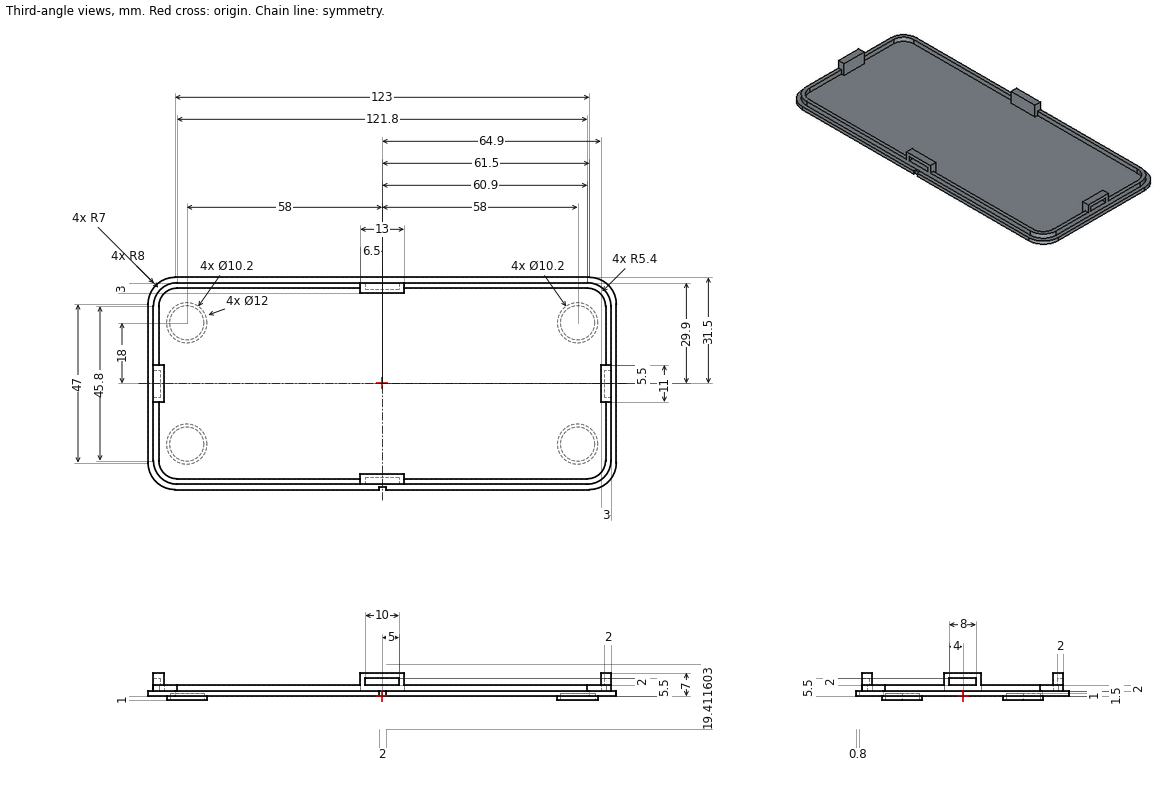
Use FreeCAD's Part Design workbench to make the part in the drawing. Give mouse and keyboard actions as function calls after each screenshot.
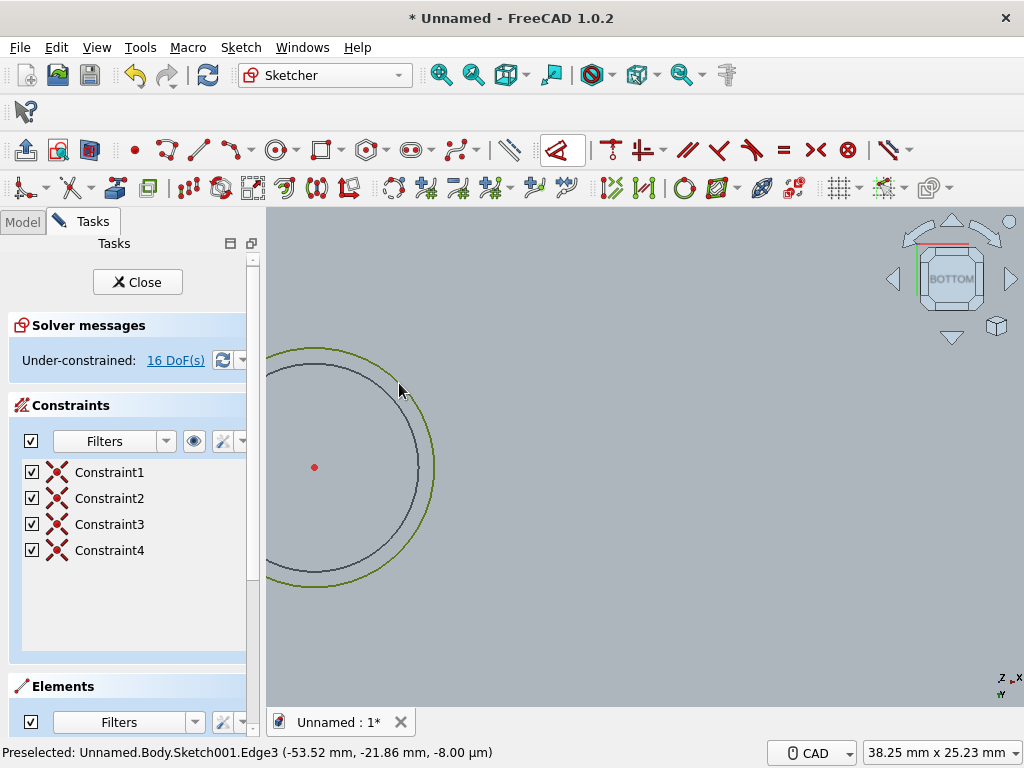
scroll(401, 385, down, 9)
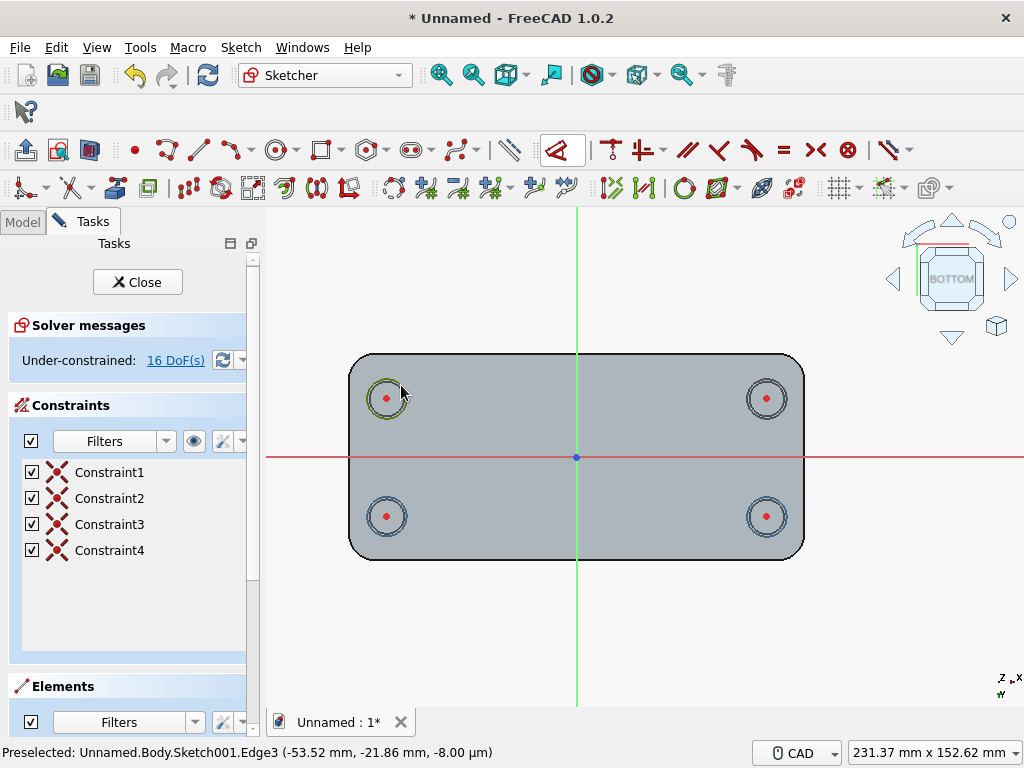
scroll(781, 385, up, 9)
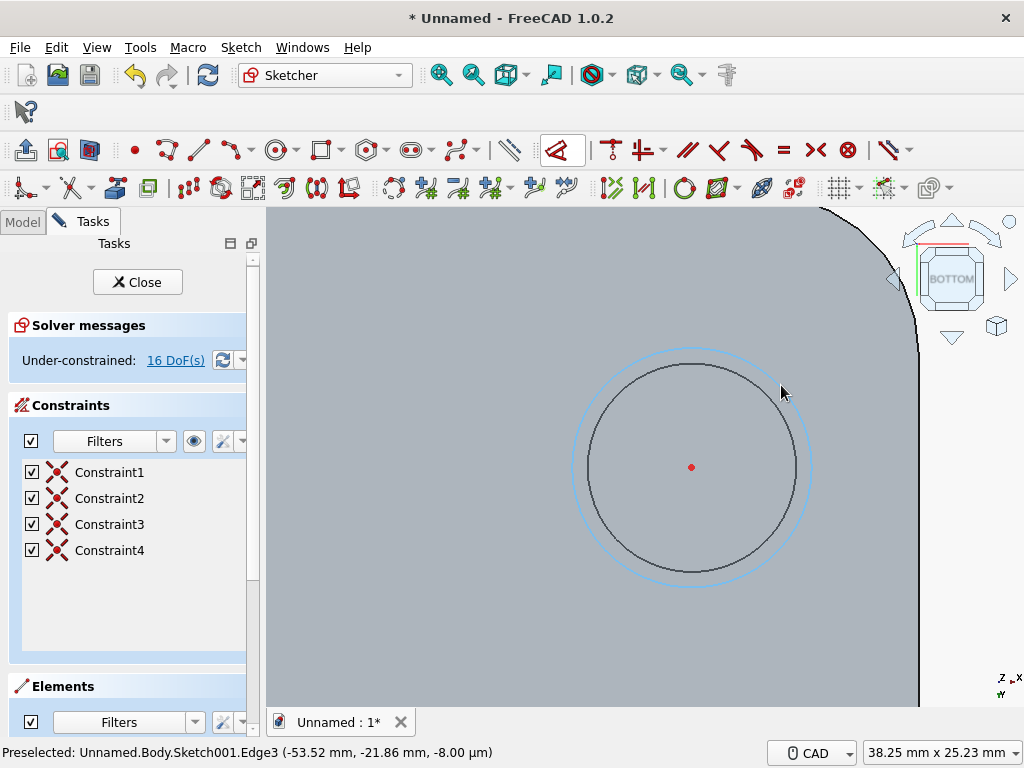
click(776, 383)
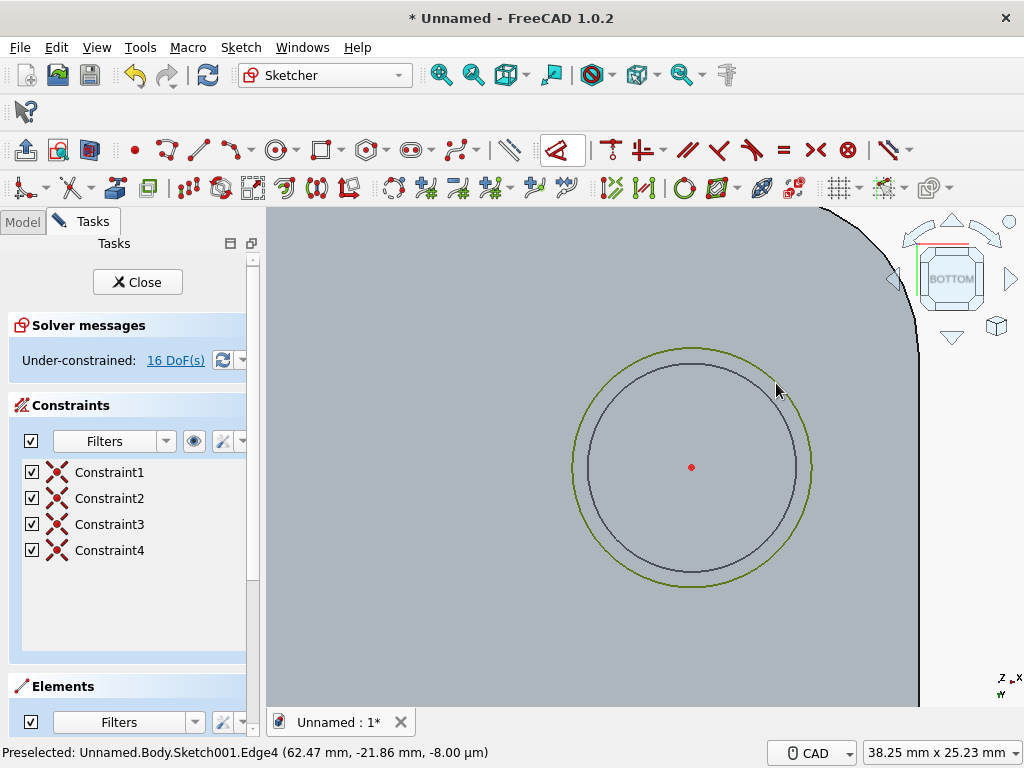
key(e)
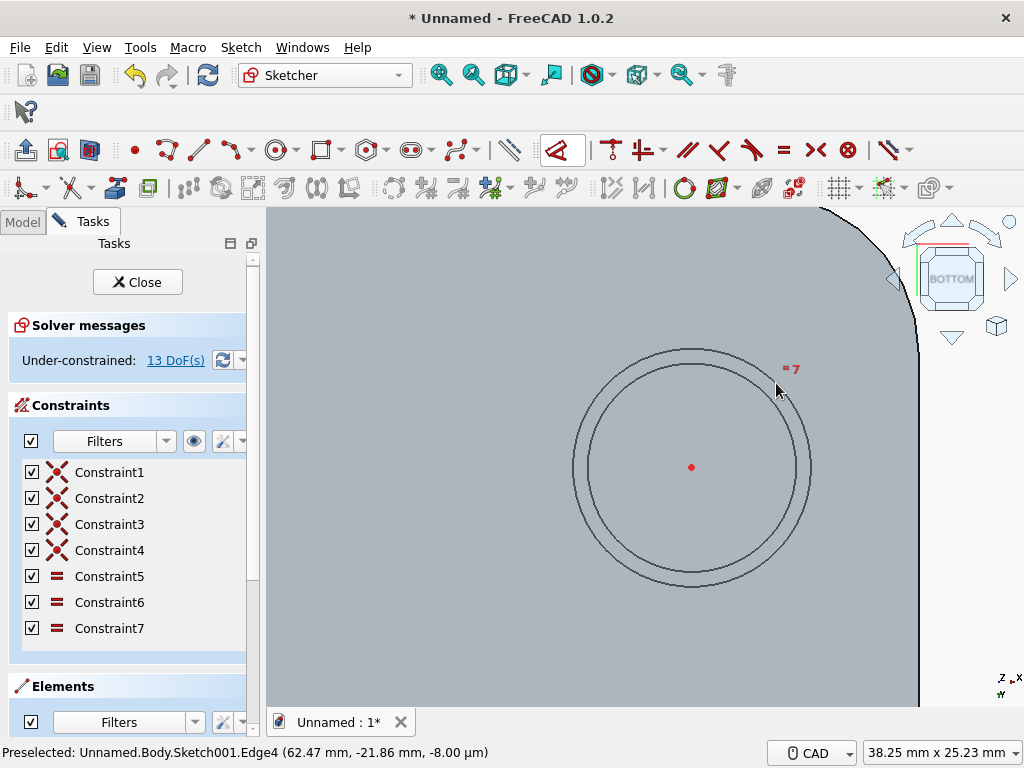
scroll(782, 385, down, 9)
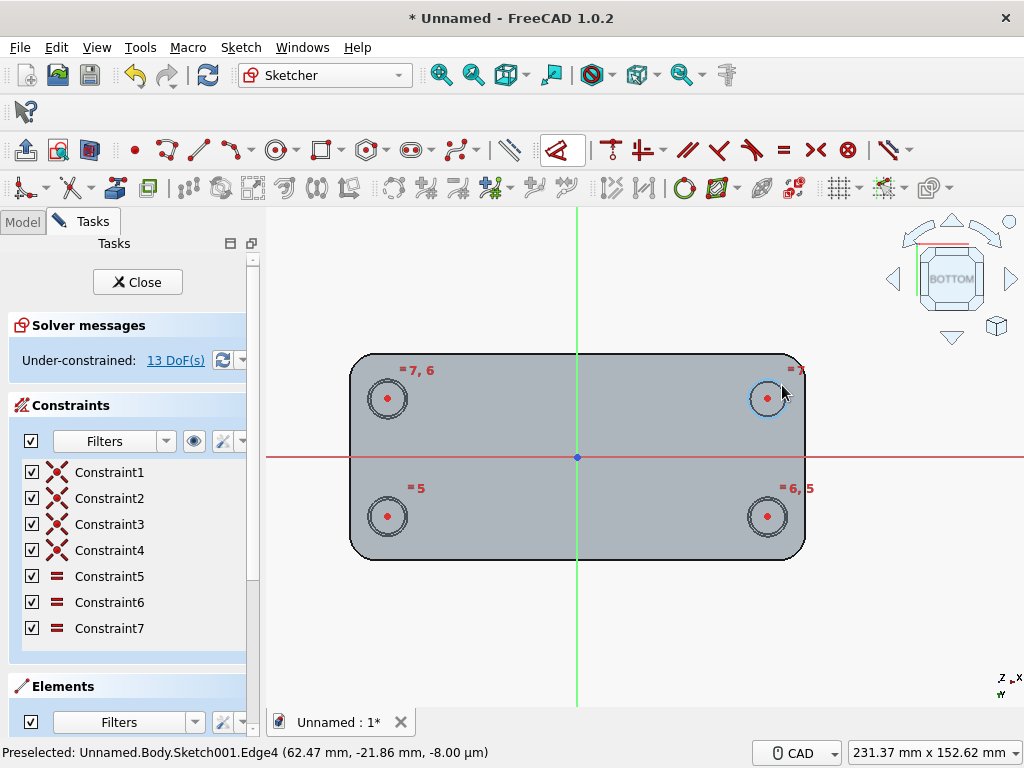
scroll(400, 504, up, 9)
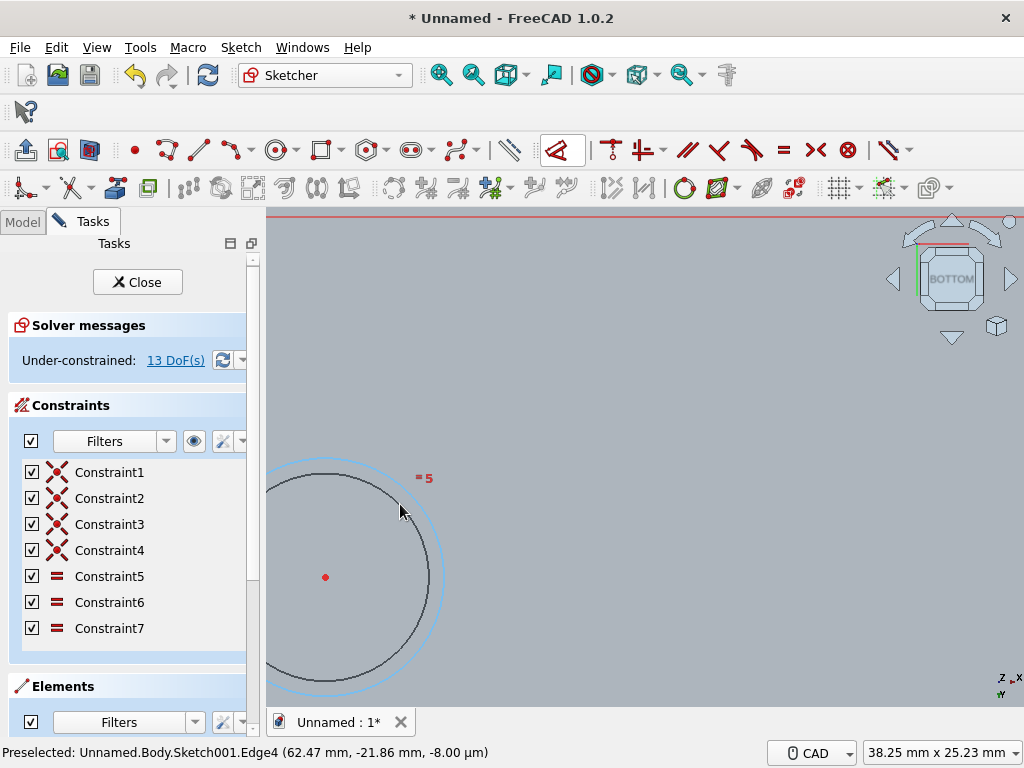
click(398, 504)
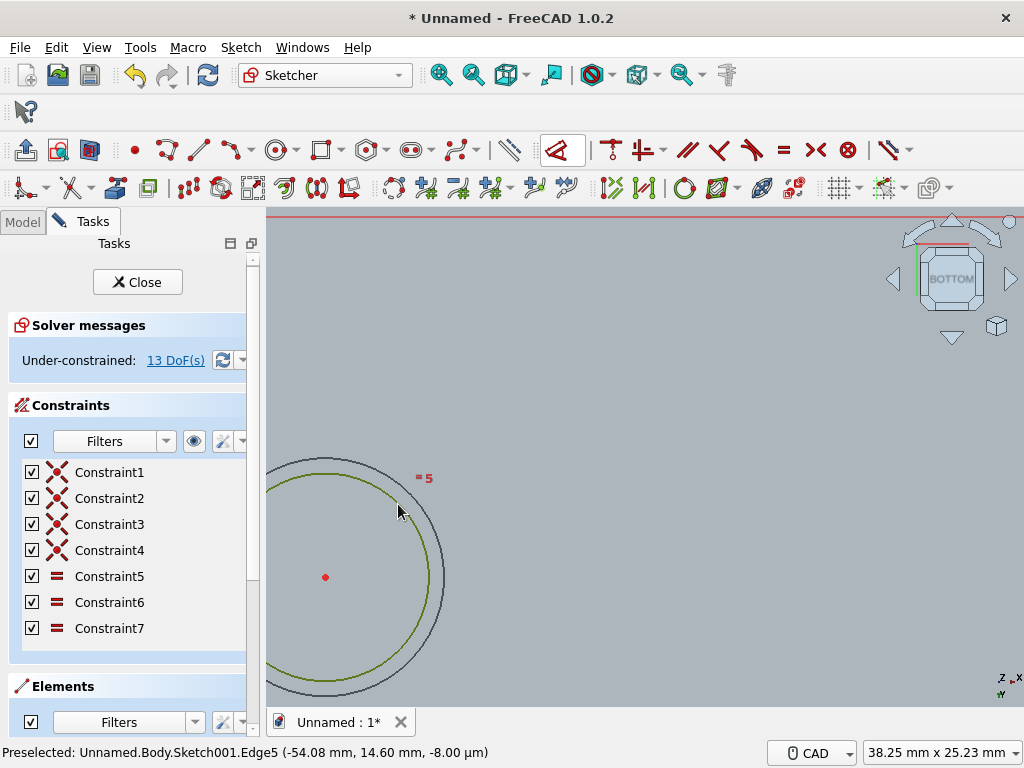
scroll(399, 505, down, 9)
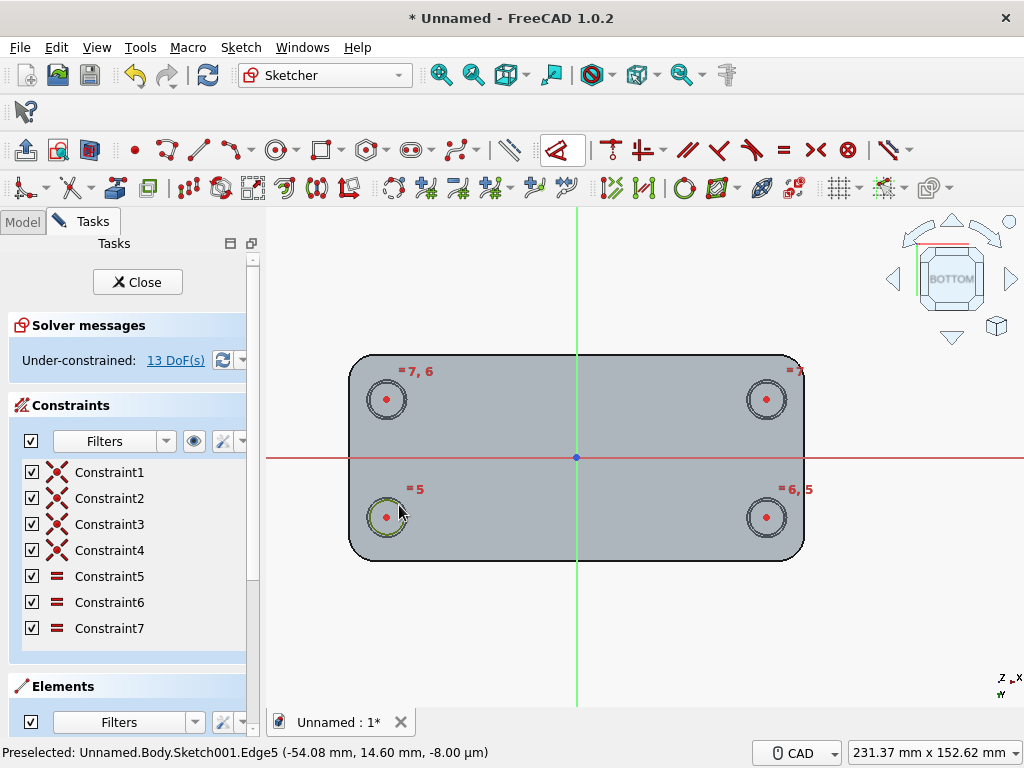
scroll(779, 506, up, 9)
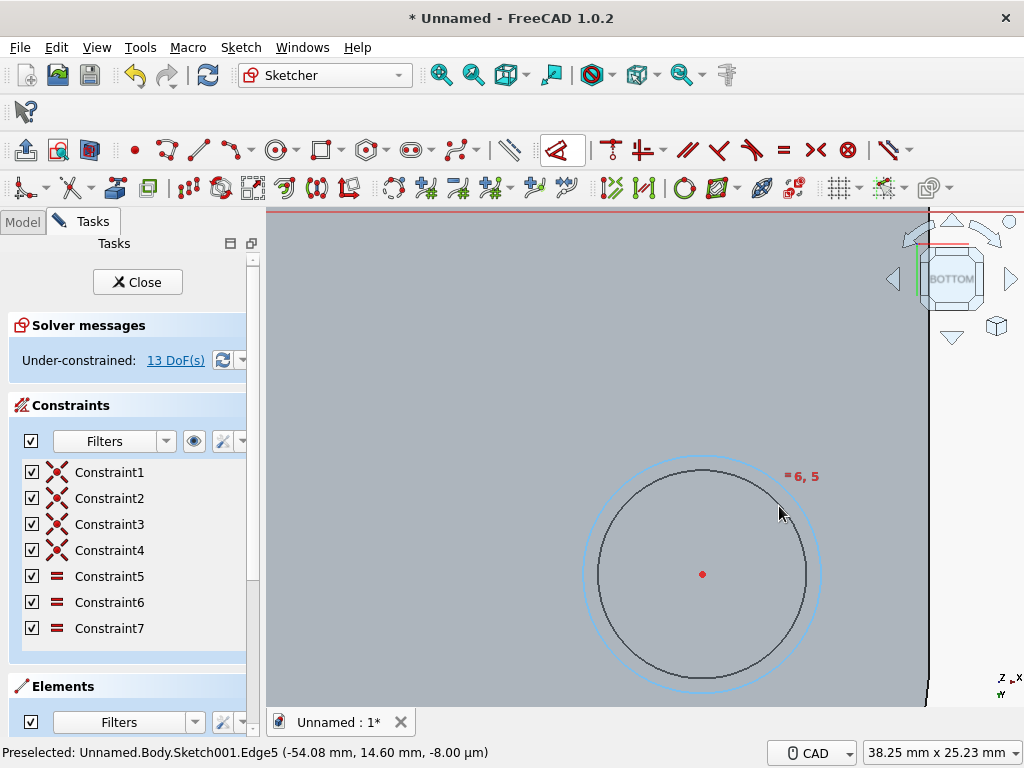
click(776, 500)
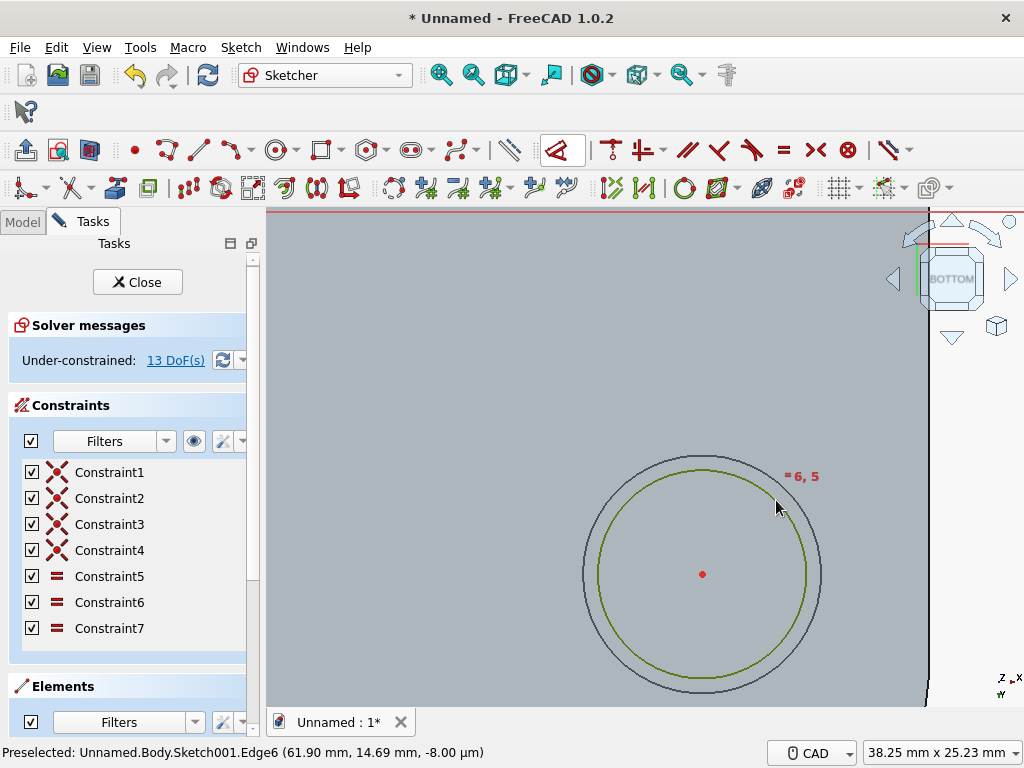
scroll(780, 506, down, 9)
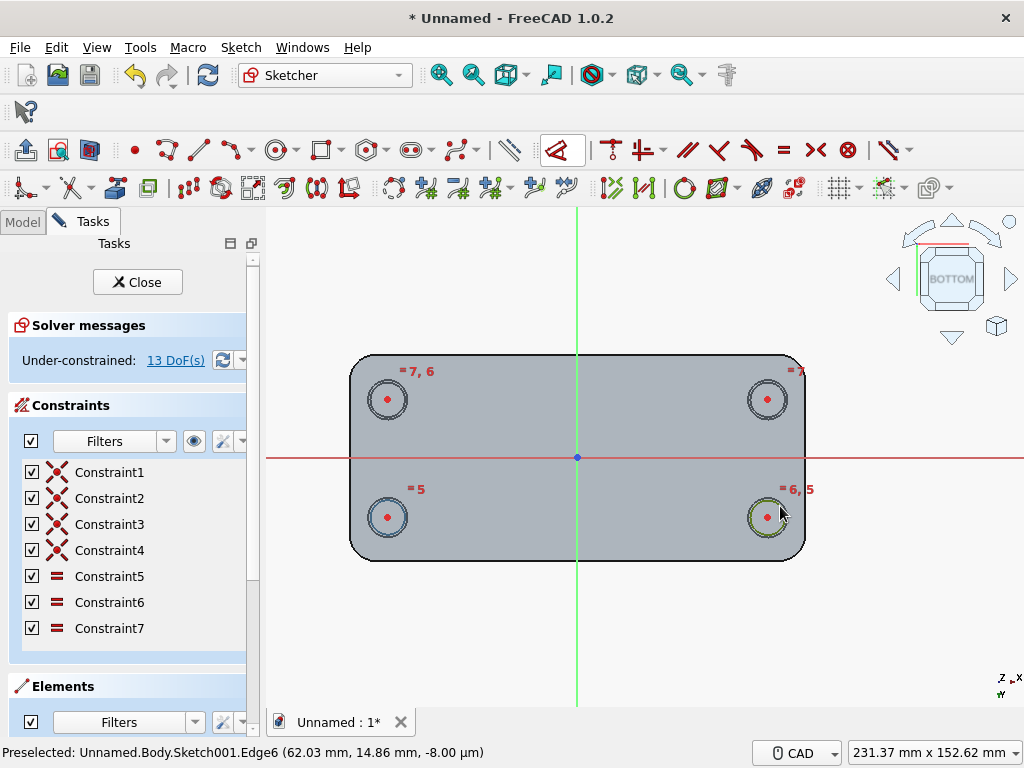
scroll(400, 388, up, 9)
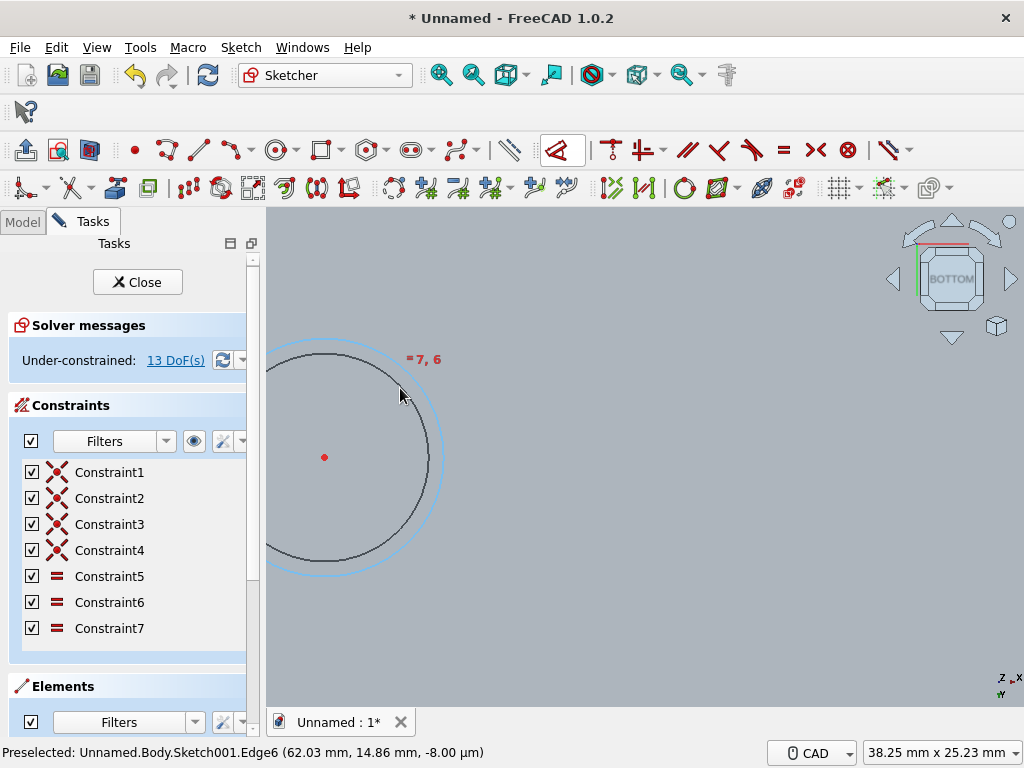
click(398, 384)